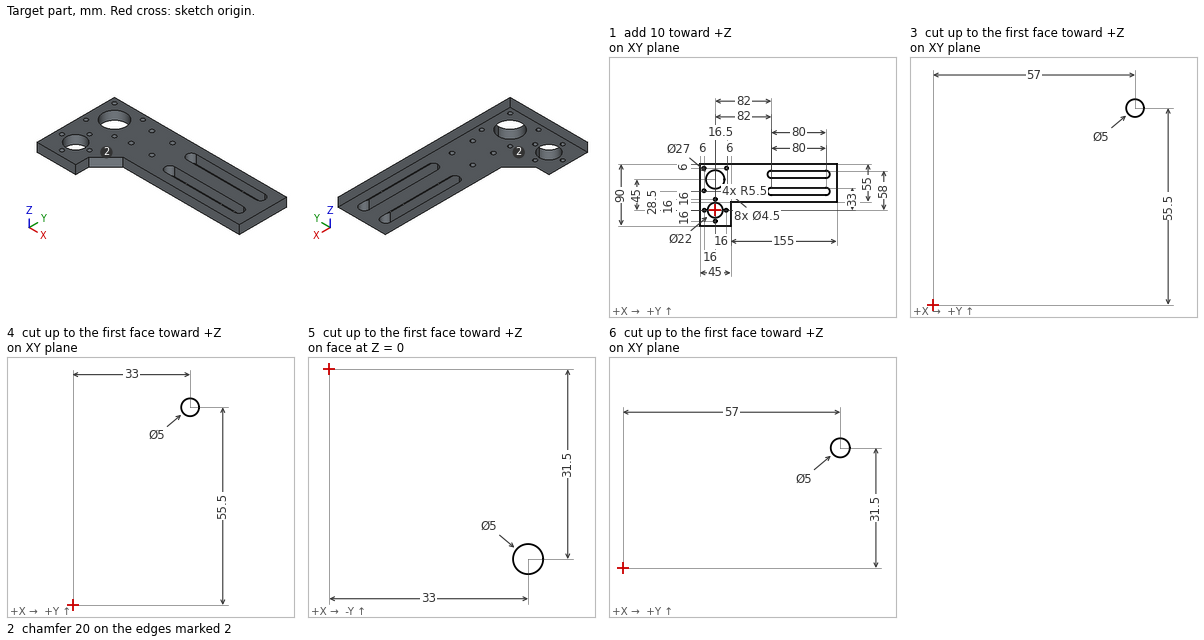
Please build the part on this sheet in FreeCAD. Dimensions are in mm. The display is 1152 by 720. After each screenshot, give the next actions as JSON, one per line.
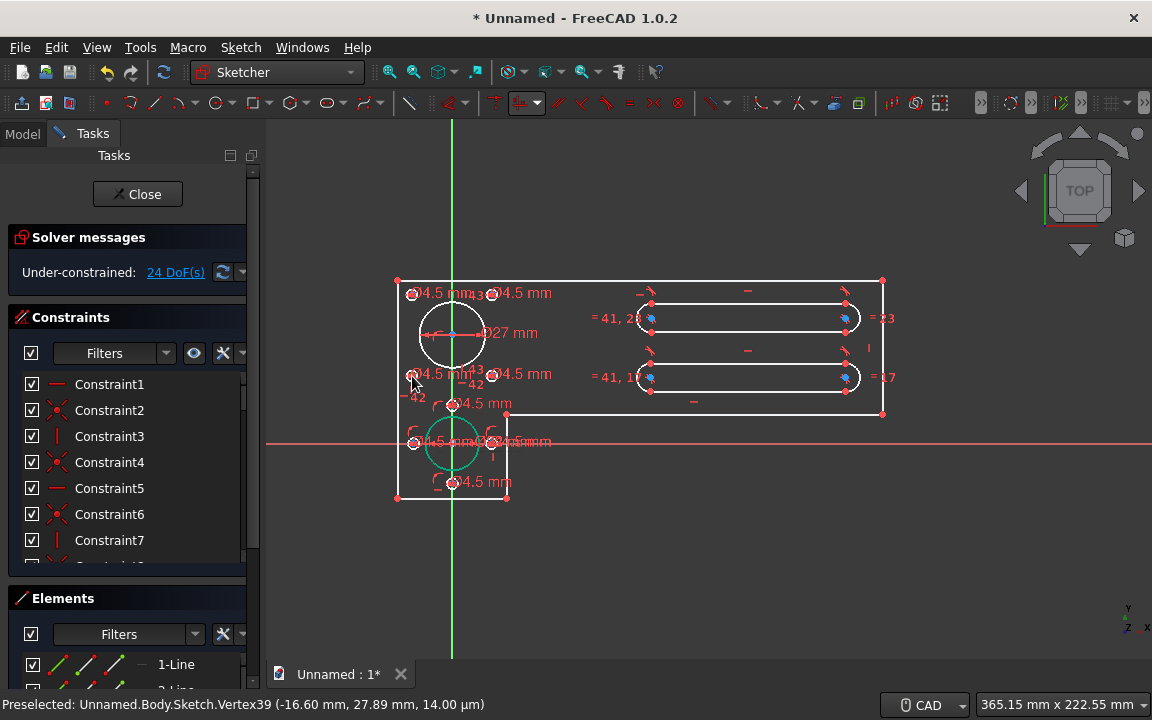
{"action": "left_click", "coordinate": [412, 295]}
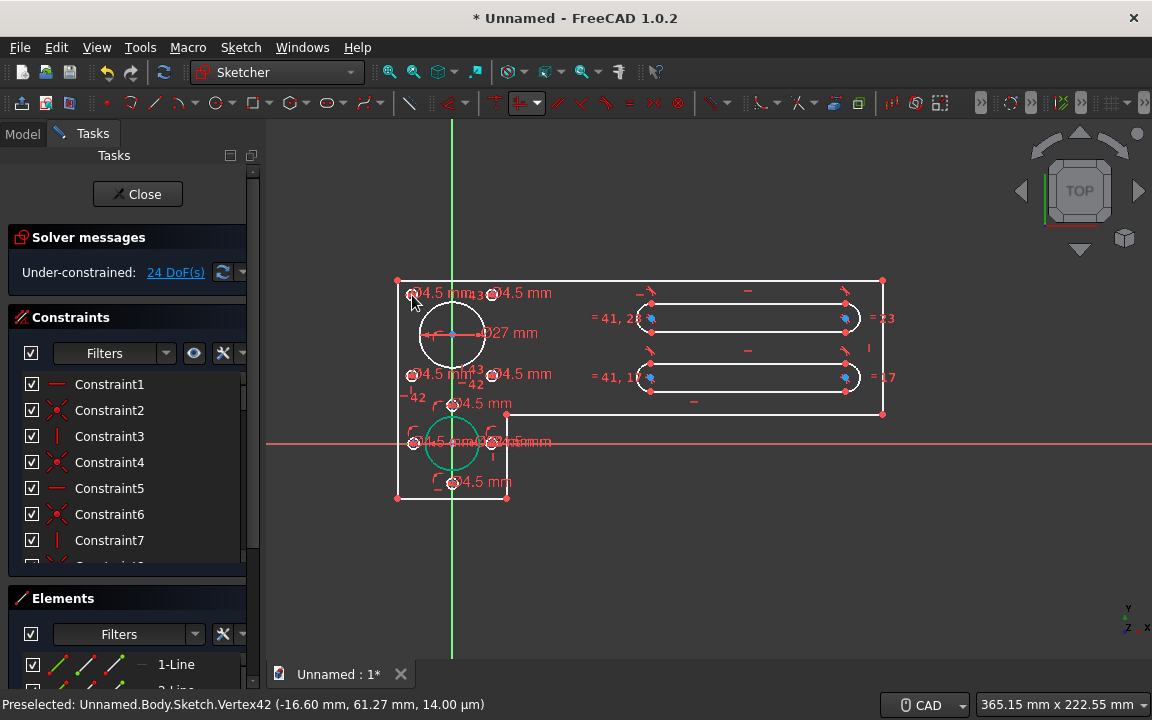
{"action": "key", "text": "v"}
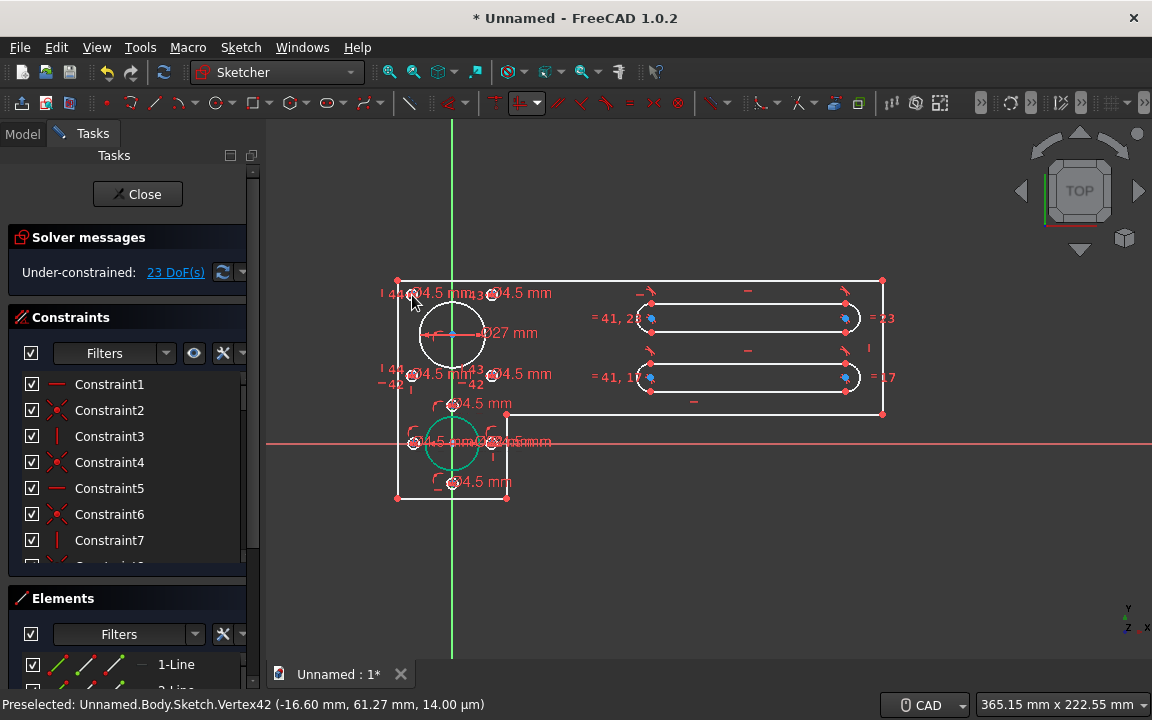
{"action": "left_click", "coordinate": [492, 295]}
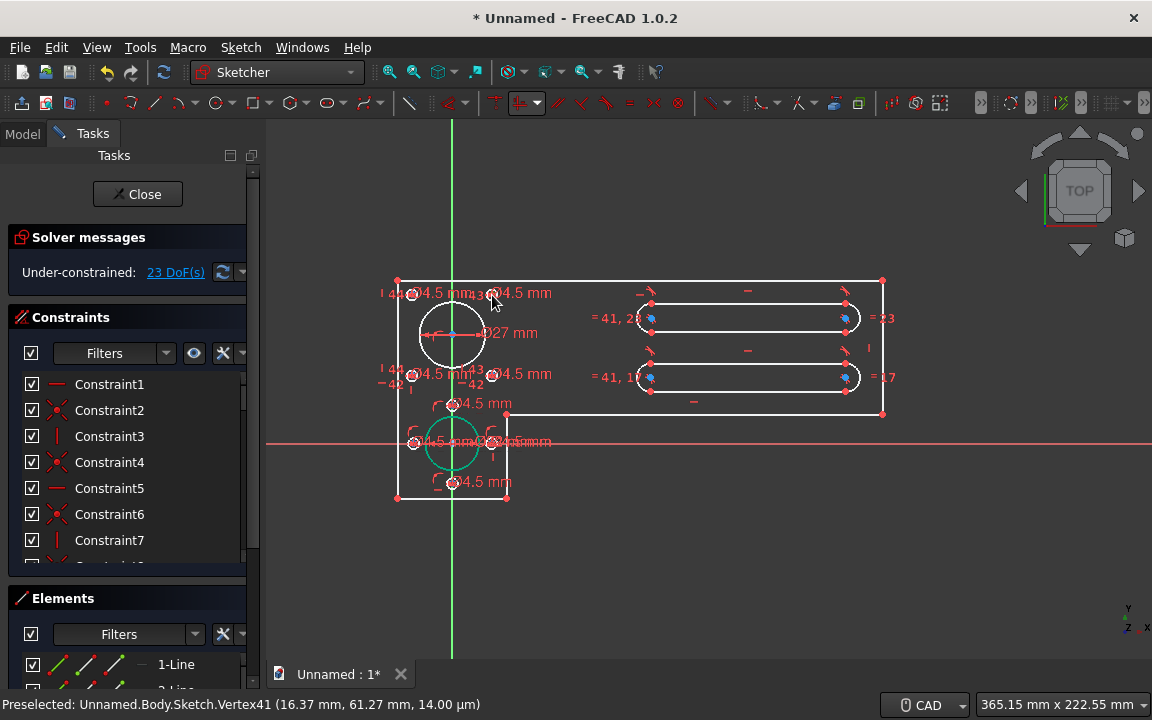
{"action": "left_click", "coordinate": [412, 295]}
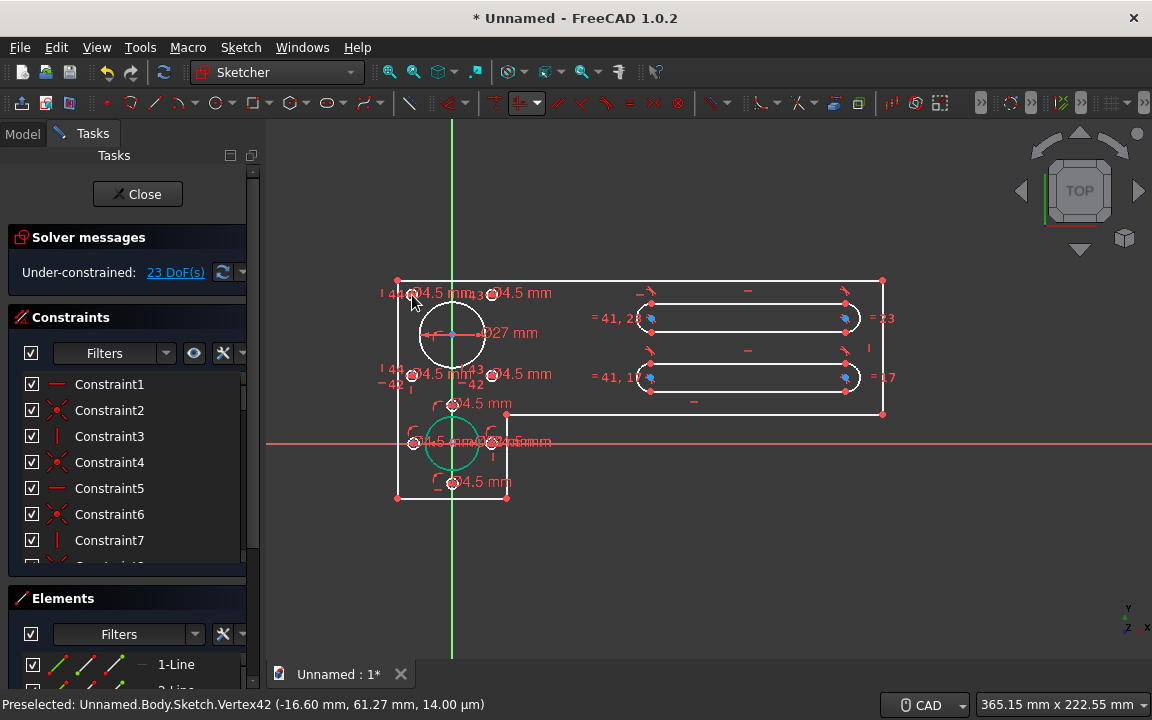
{"action": "key", "text": "h"}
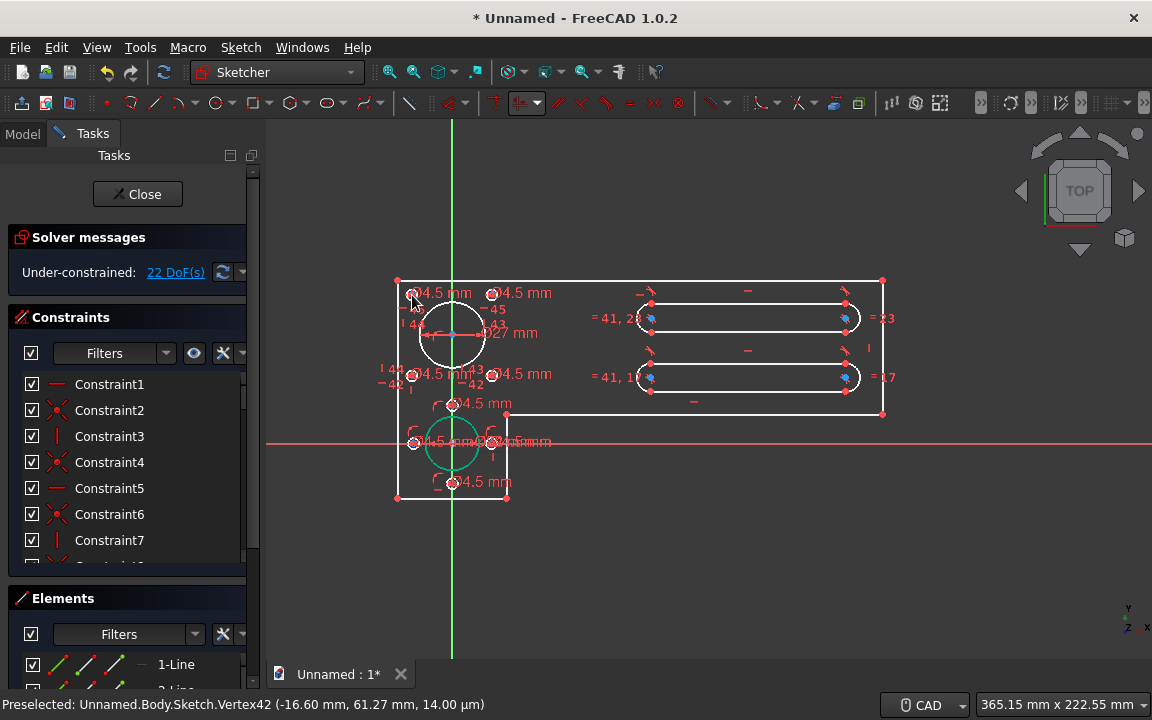
{"action": "left_click", "coordinate": [448, 104]}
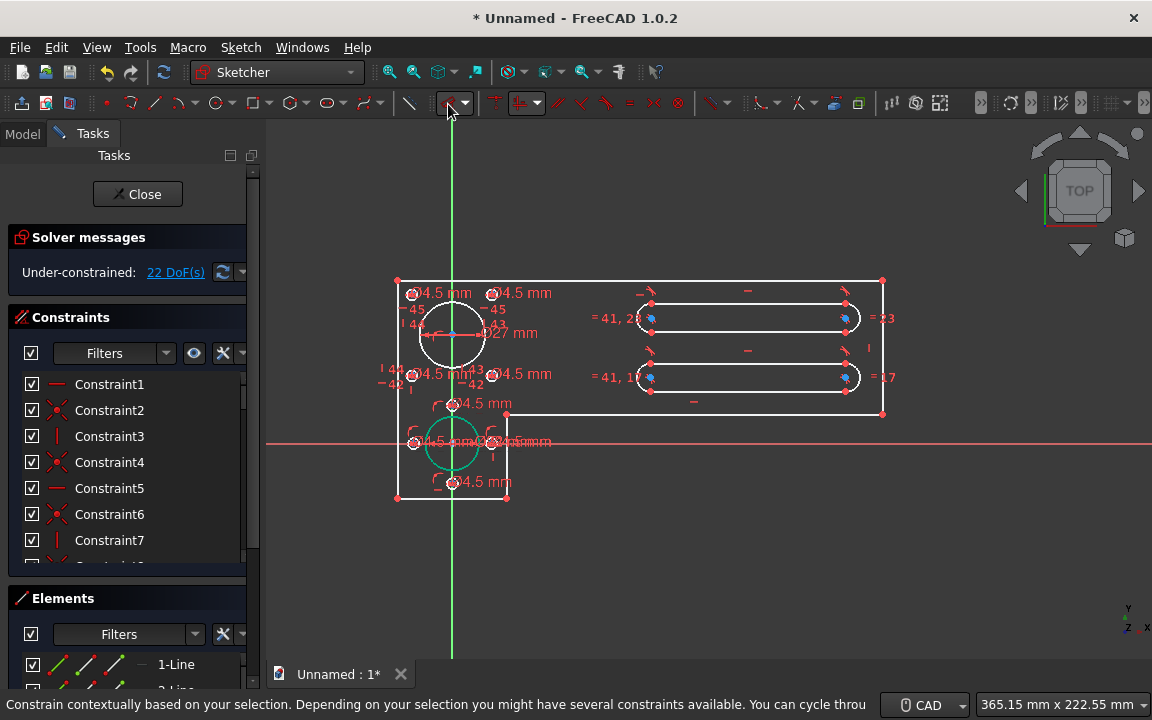
{"action": "scroll", "coordinate": [640, 369], "scroll_direction": "up", "scroll_amount": 6}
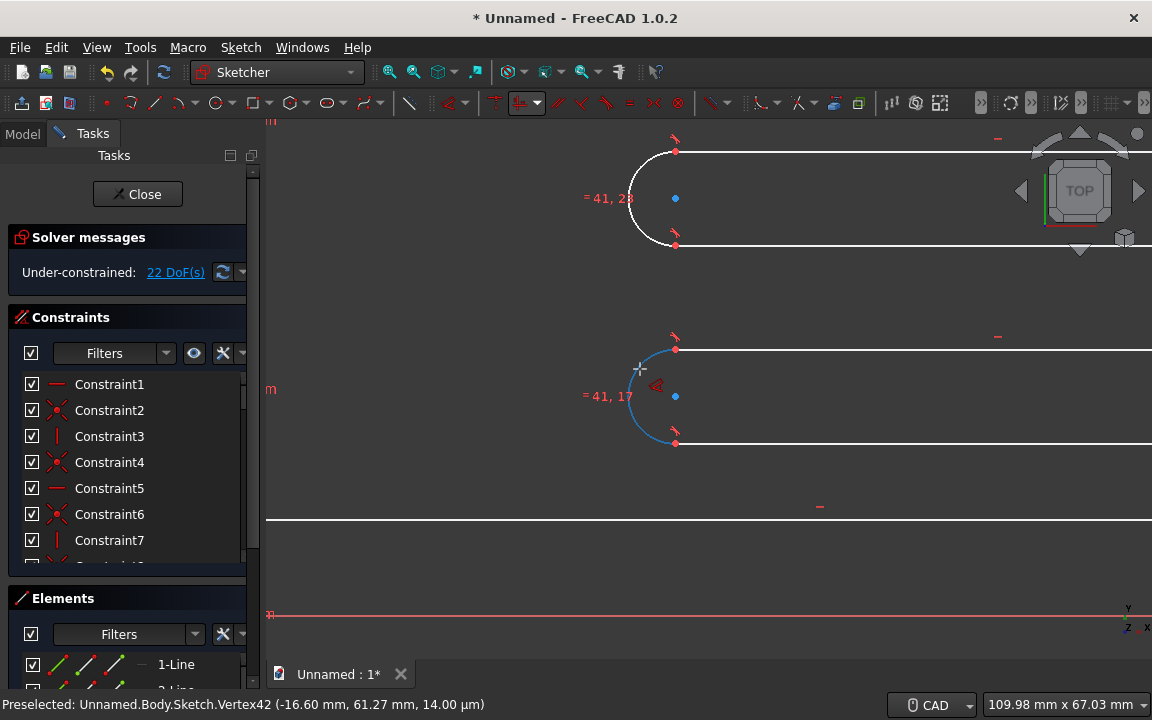
{"action": "left_click", "coordinate": [637, 369]}
{"action": "left_click", "coordinate": [611, 350]}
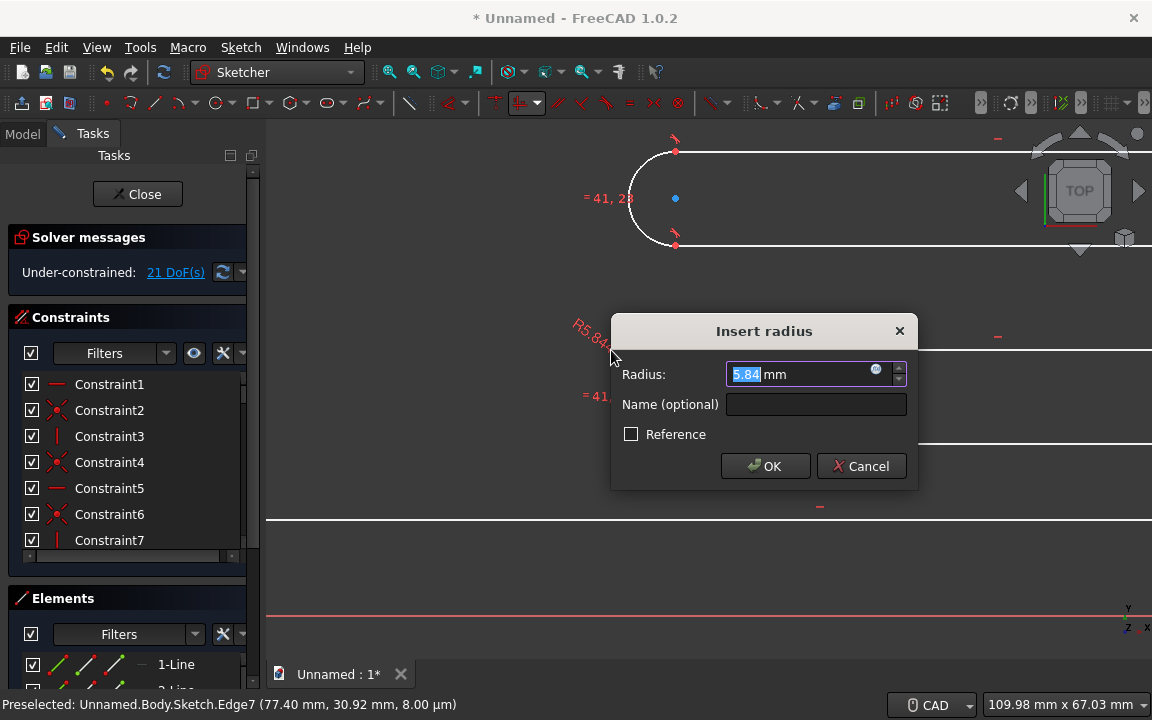
{"action": "type", "text": "5.5"}
{"action": "key", "text": "Return"}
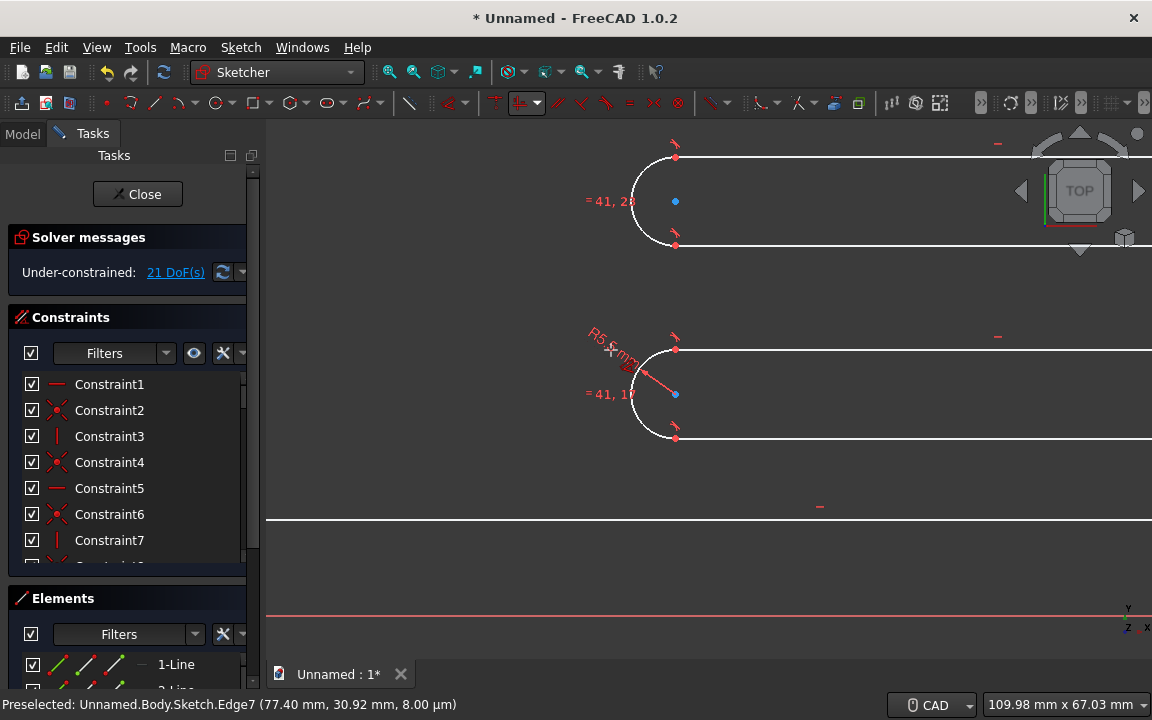
{"action": "scroll", "coordinate": [641, 369], "scroll_direction": "down", "scroll_amount": 6}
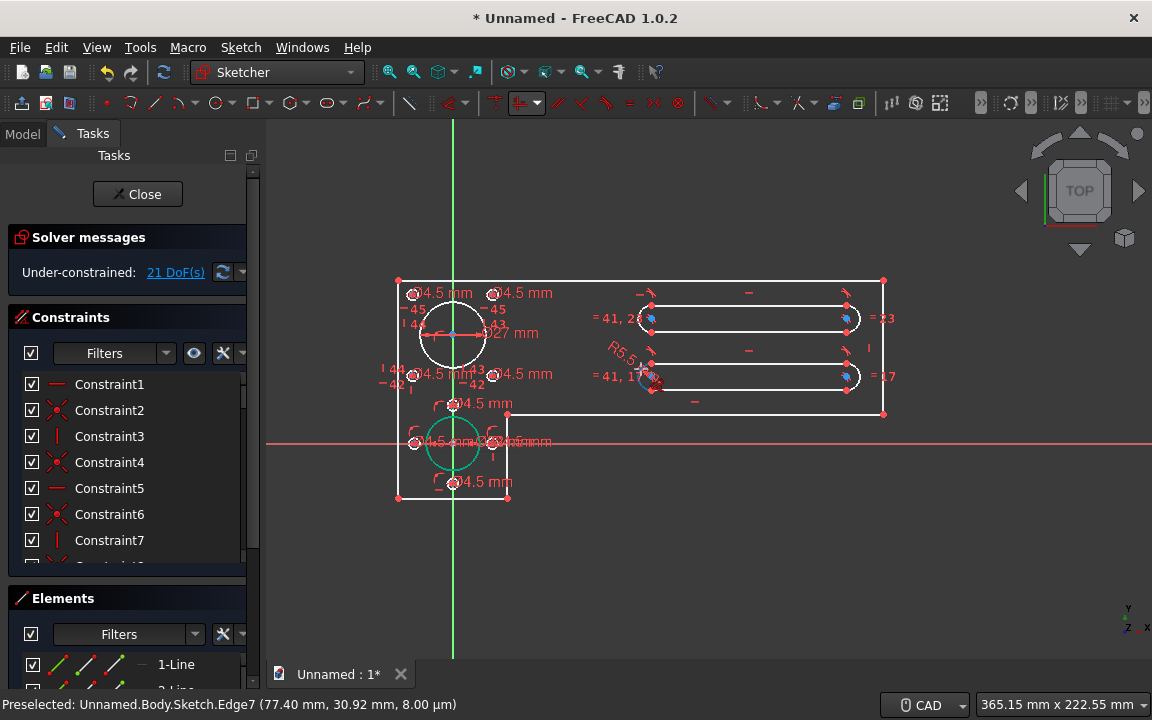
{"action": "left_click", "coordinate": [883, 375]}
{"action": "left_click", "coordinate": [917, 348]}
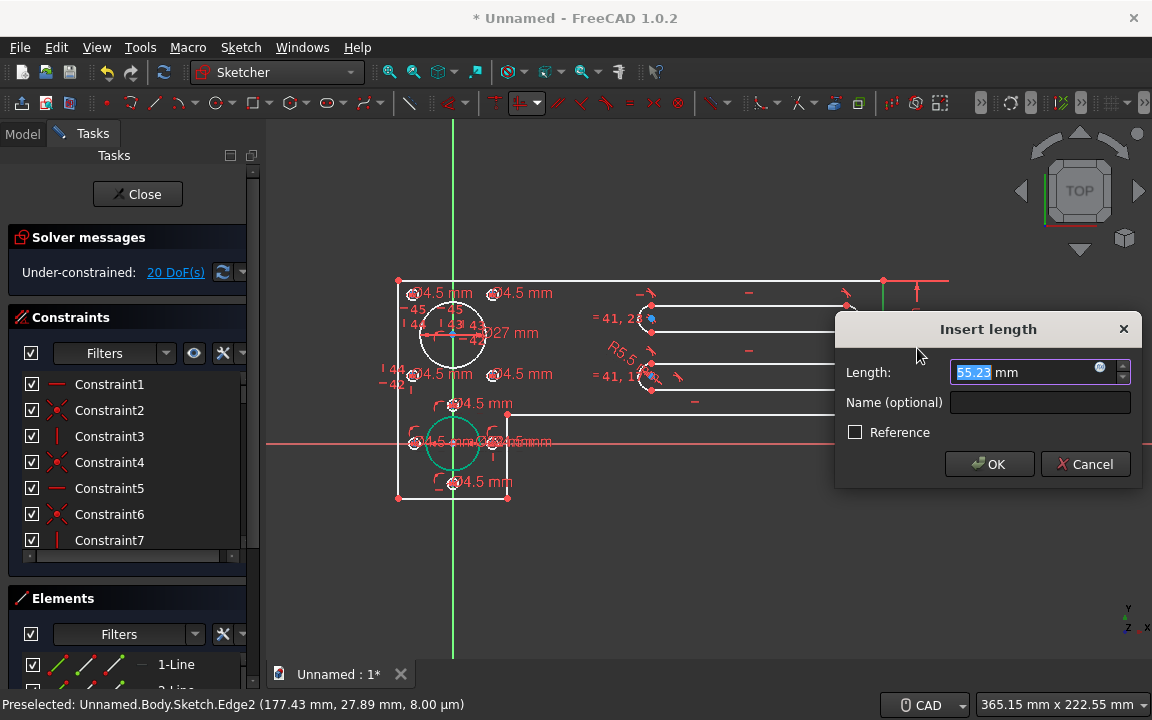
{"action": "type", "text": "55"}
{"action": "key", "text": "Return"}